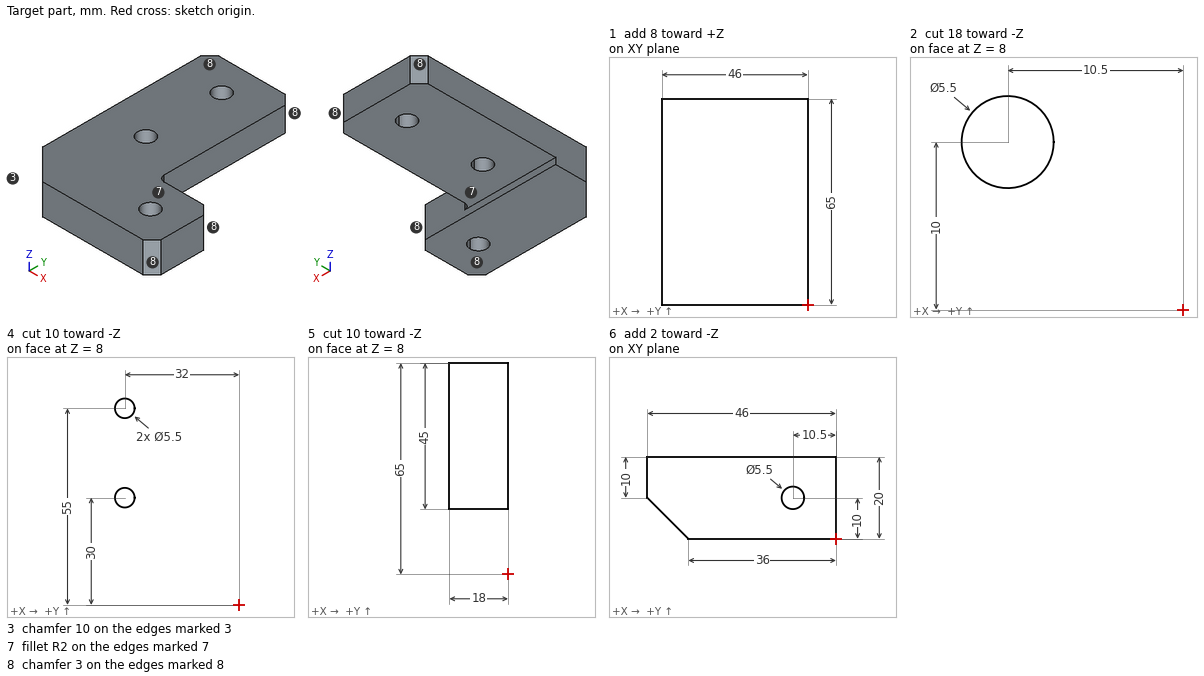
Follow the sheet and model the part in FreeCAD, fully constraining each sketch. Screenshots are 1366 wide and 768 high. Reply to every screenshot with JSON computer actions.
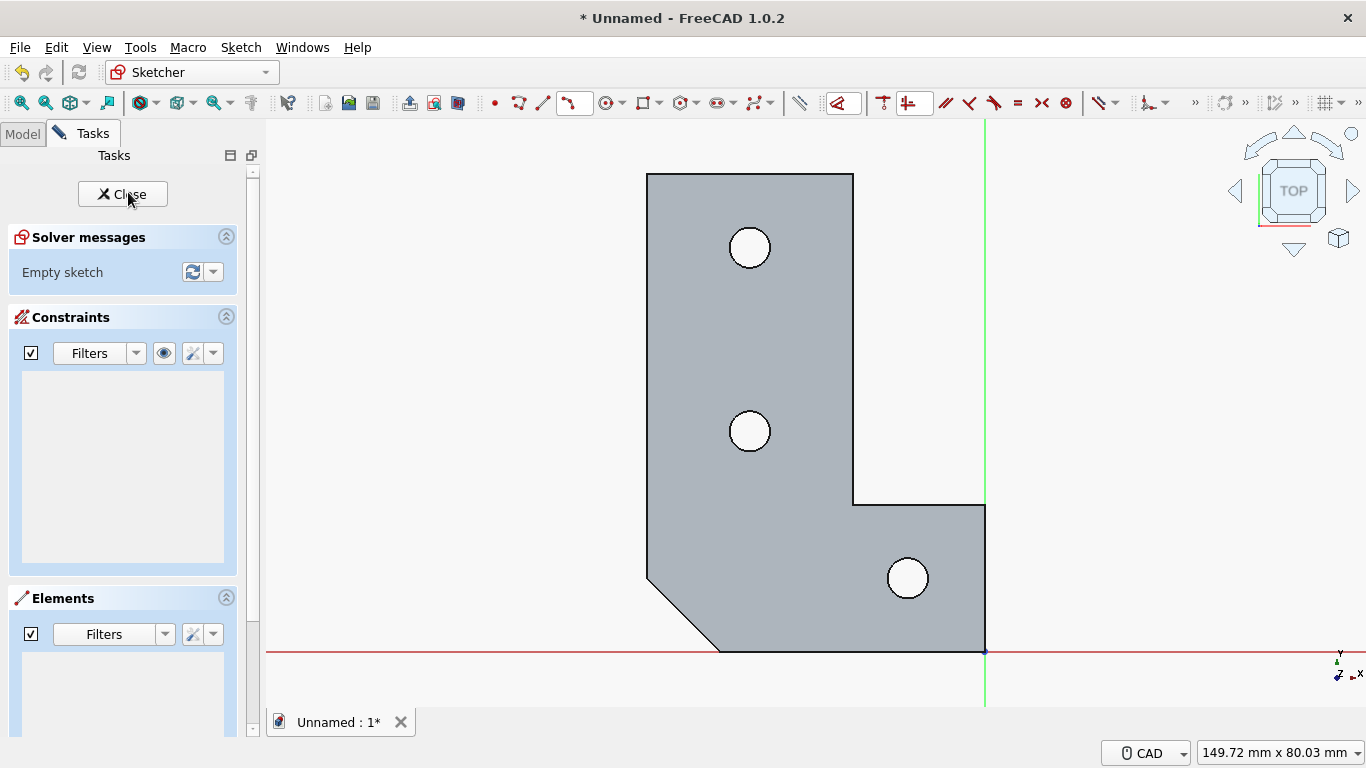
{"action": "left_click", "coordinate": [458, 104]}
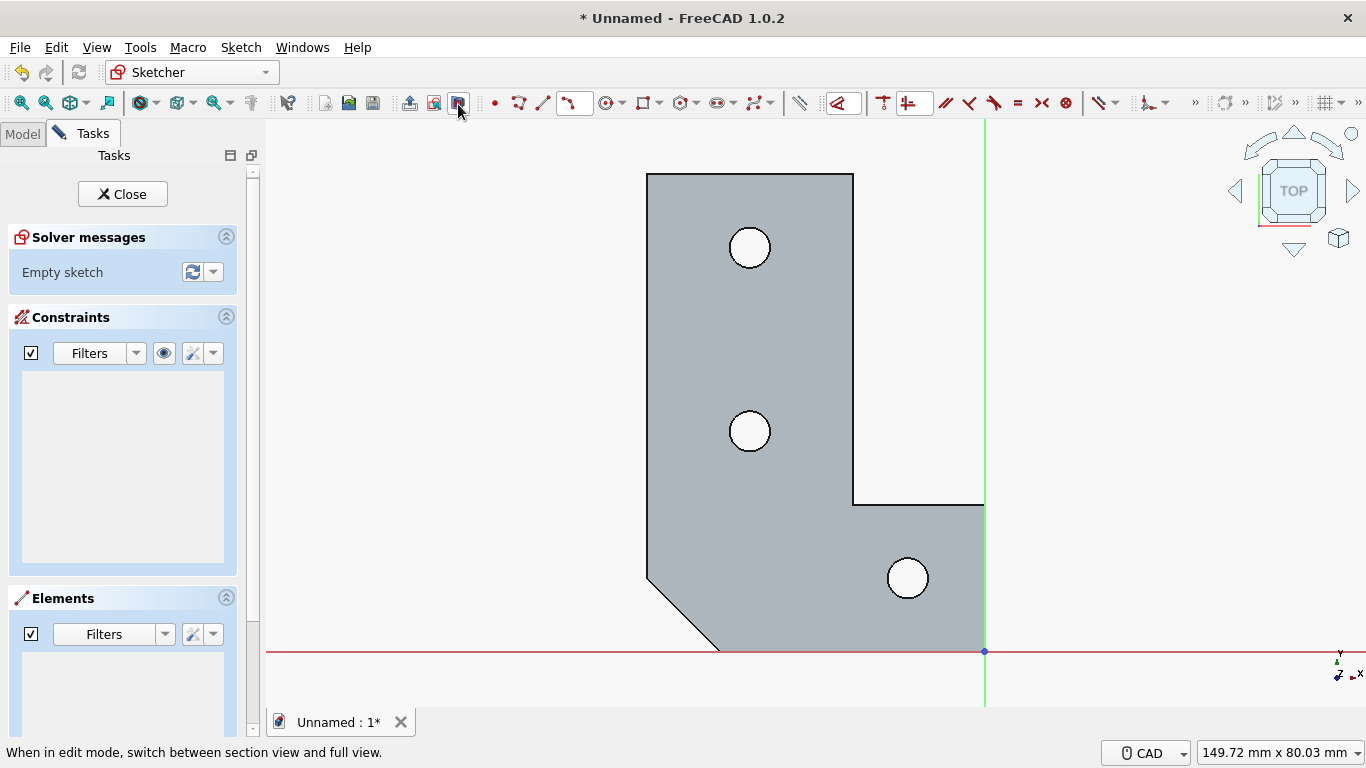
{"action": "scroll", "coordinate": [899, 679], "scroll_direction": "up", "scroll_amount": 3}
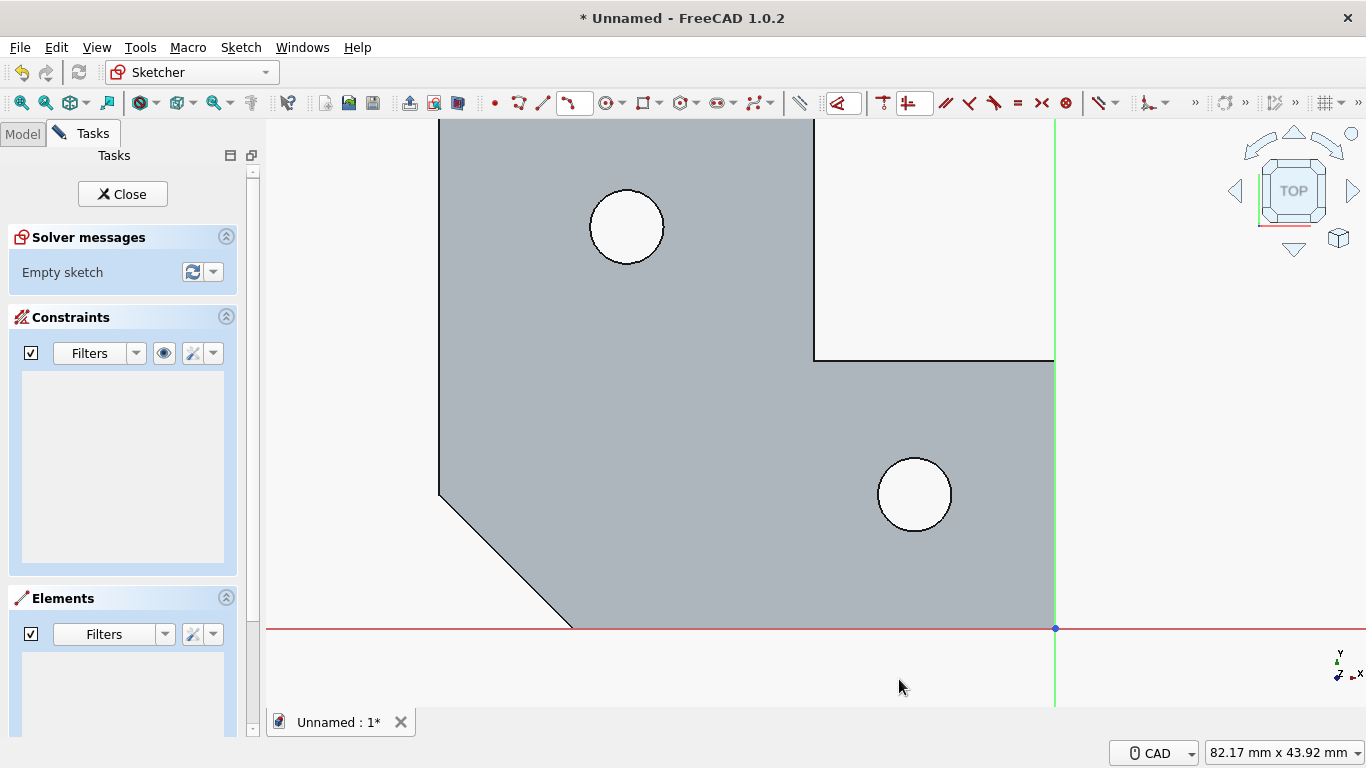
{"action": "left_click", "coordinate": [520, 104]}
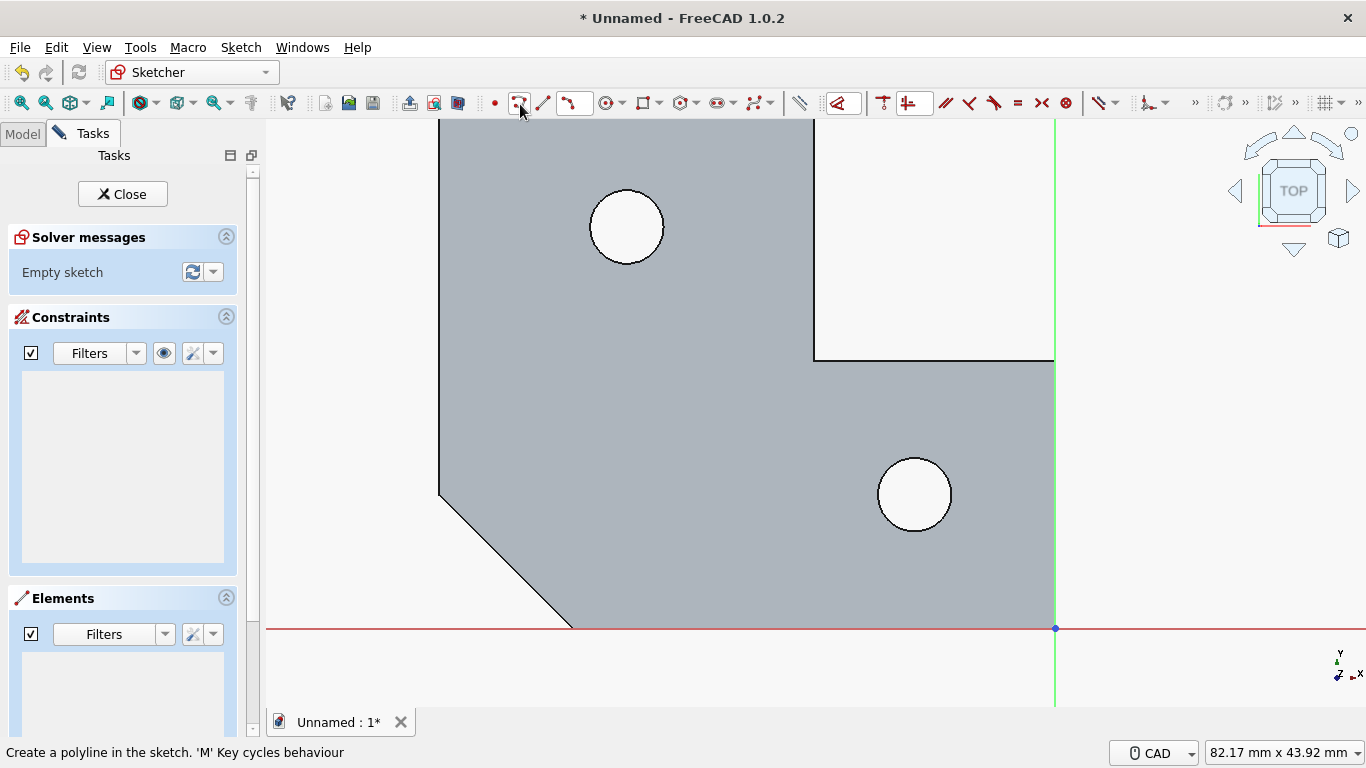
{"action": "left_click", "coordinate": [1055, 629]}
{"action": "left_click", "coordinate": [573, 620]}
{"action": "left_click", "coordinate": [439, 495]}
{"action": "left_click", "coordinate": [439, 361]}
{"action": "left_click", "coordinate": [1046, 361]}
{"action": "left_click", "coordinate": [1055, 629]}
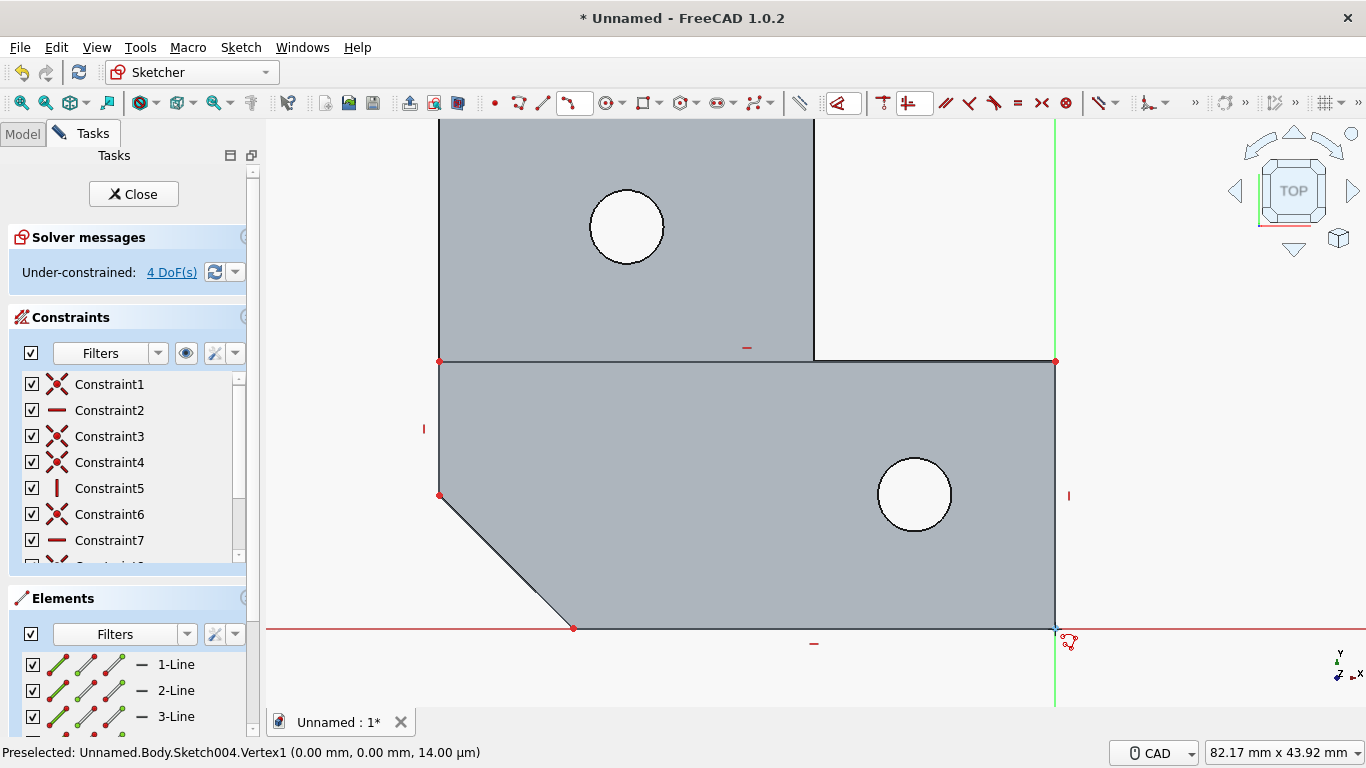
{"action": "key", "text": "g c"}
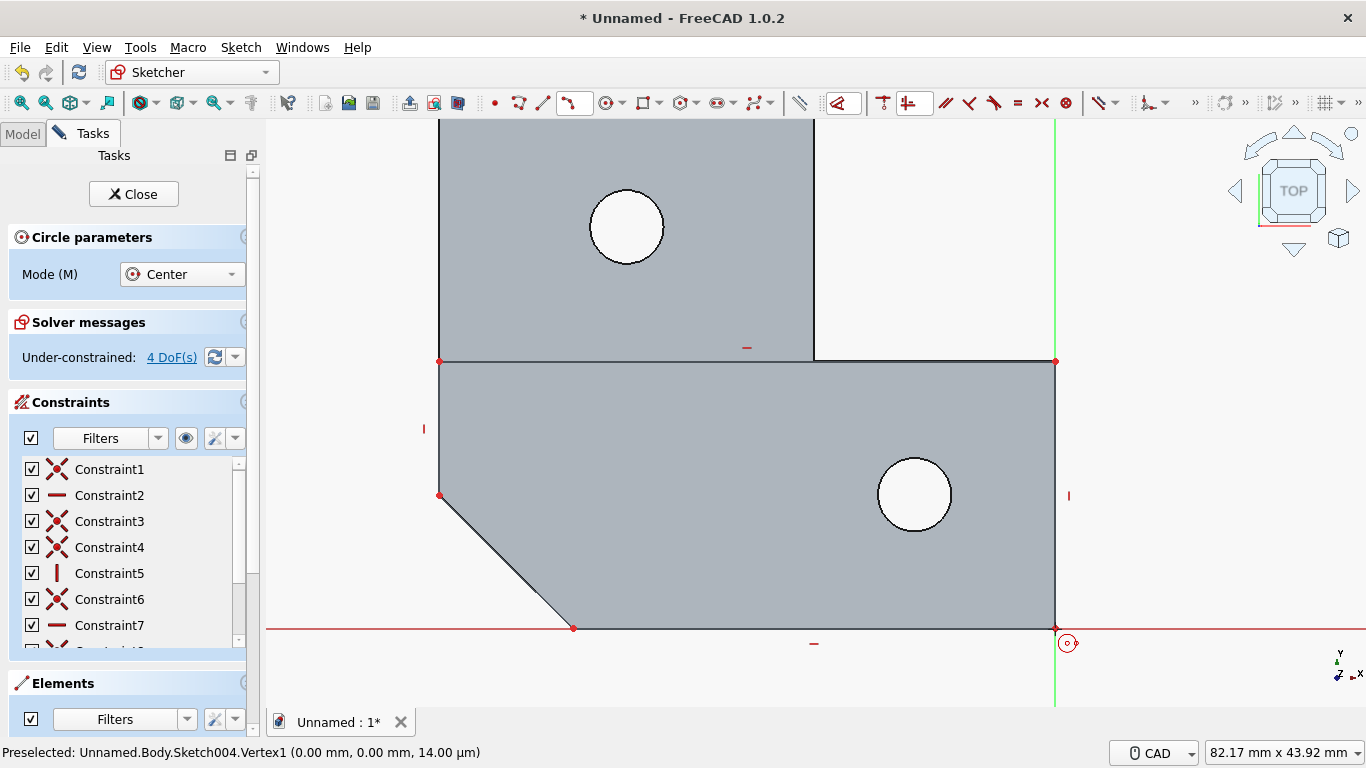
{"action": "left_click", "coordinate": [915, 495]}
{"action": "left_click", "coordinate": [941, 469]}
{"action": "key", "text": "Escape"}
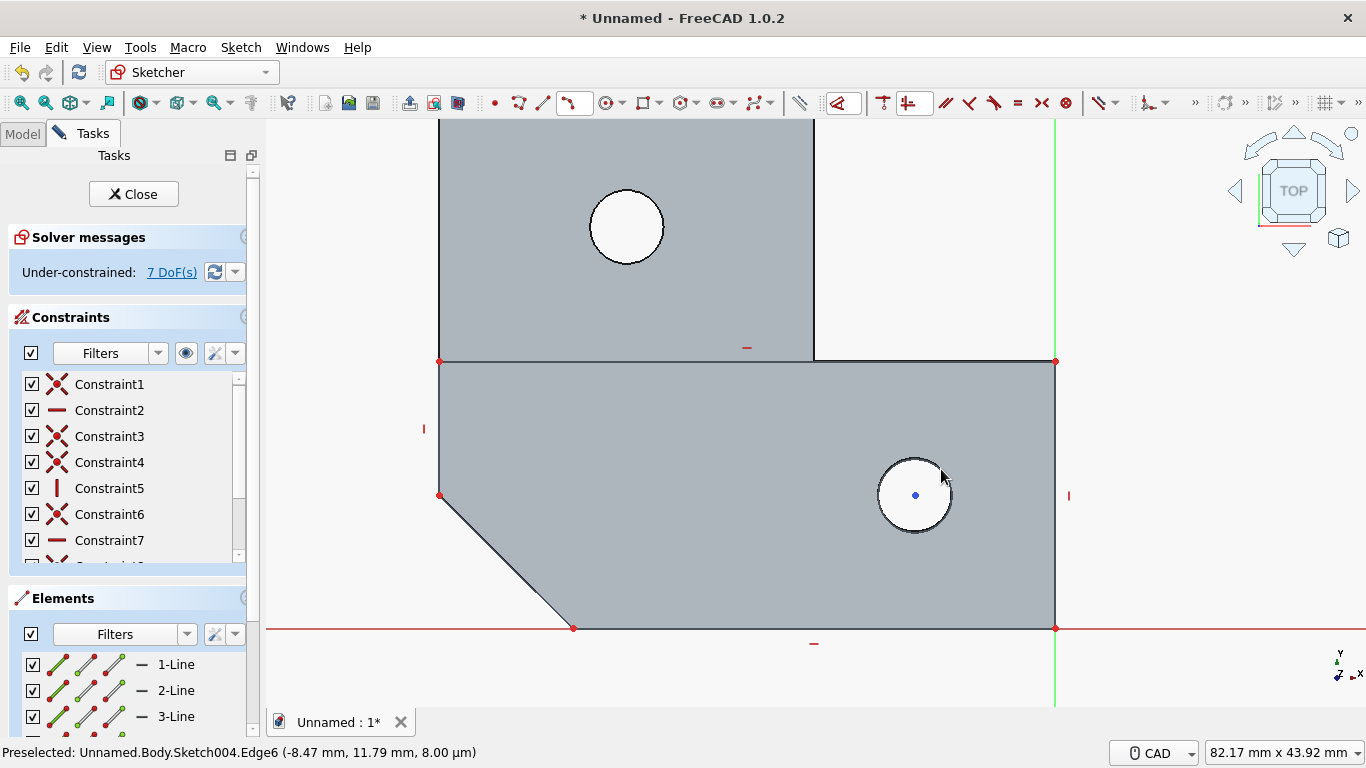
{"action": "left_click", "coordinate": [941, 470]}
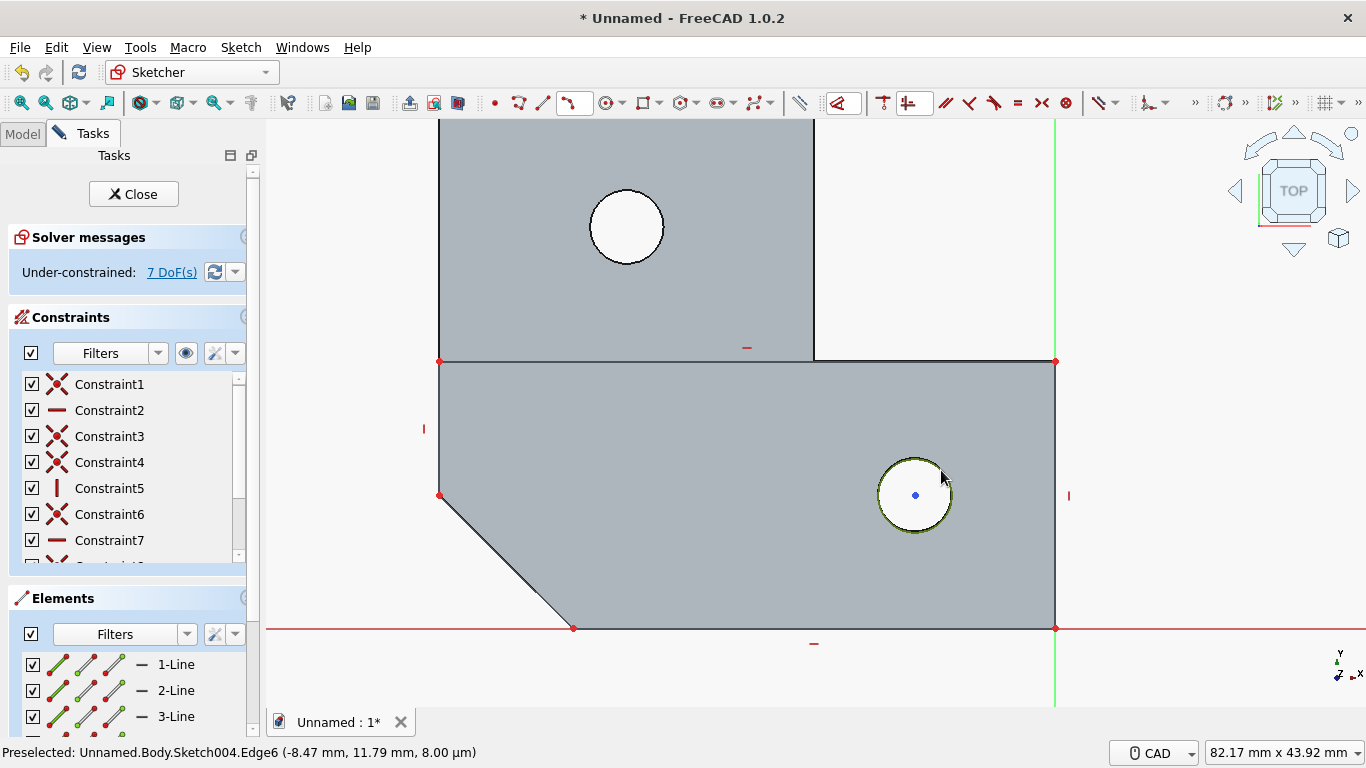
{"action": "left_click", "coordinate": [856, 104]}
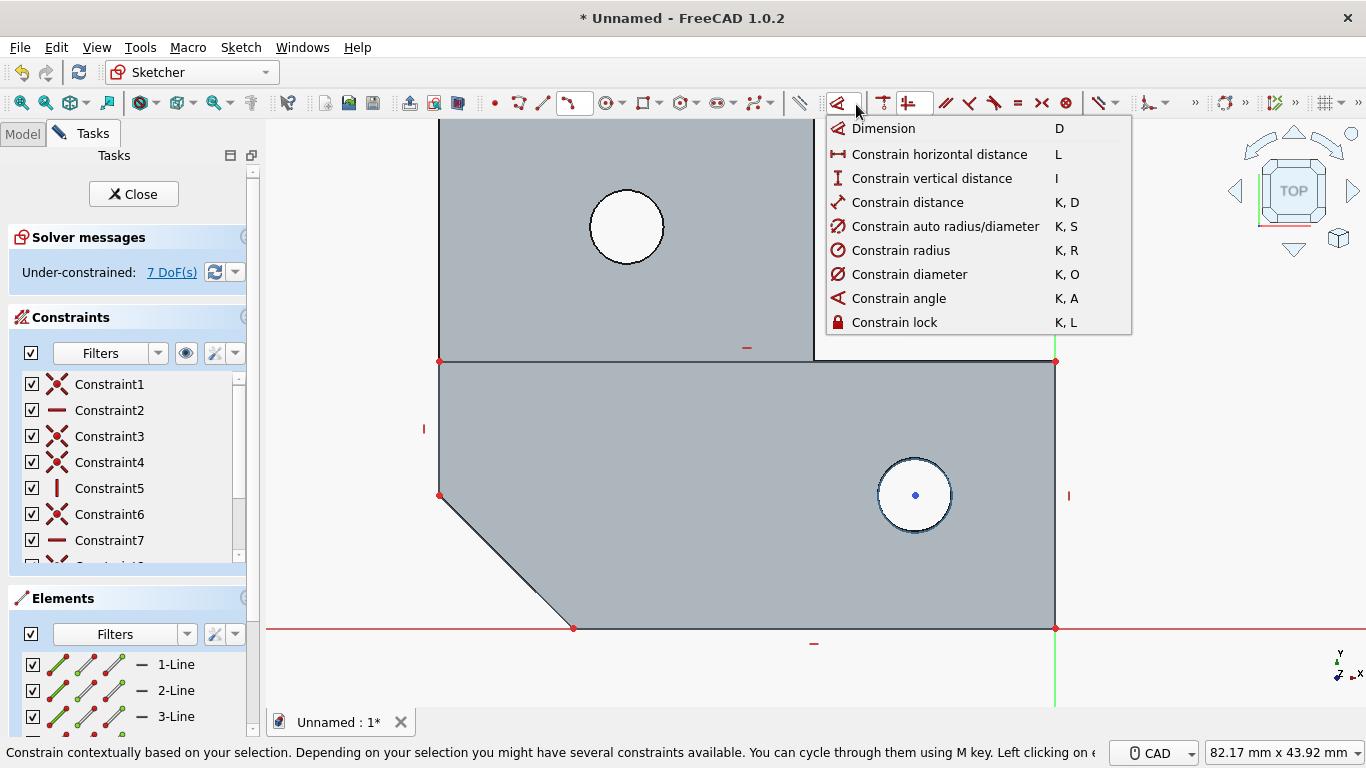
{"action": "left_click", "coordinate": [979, 274]}